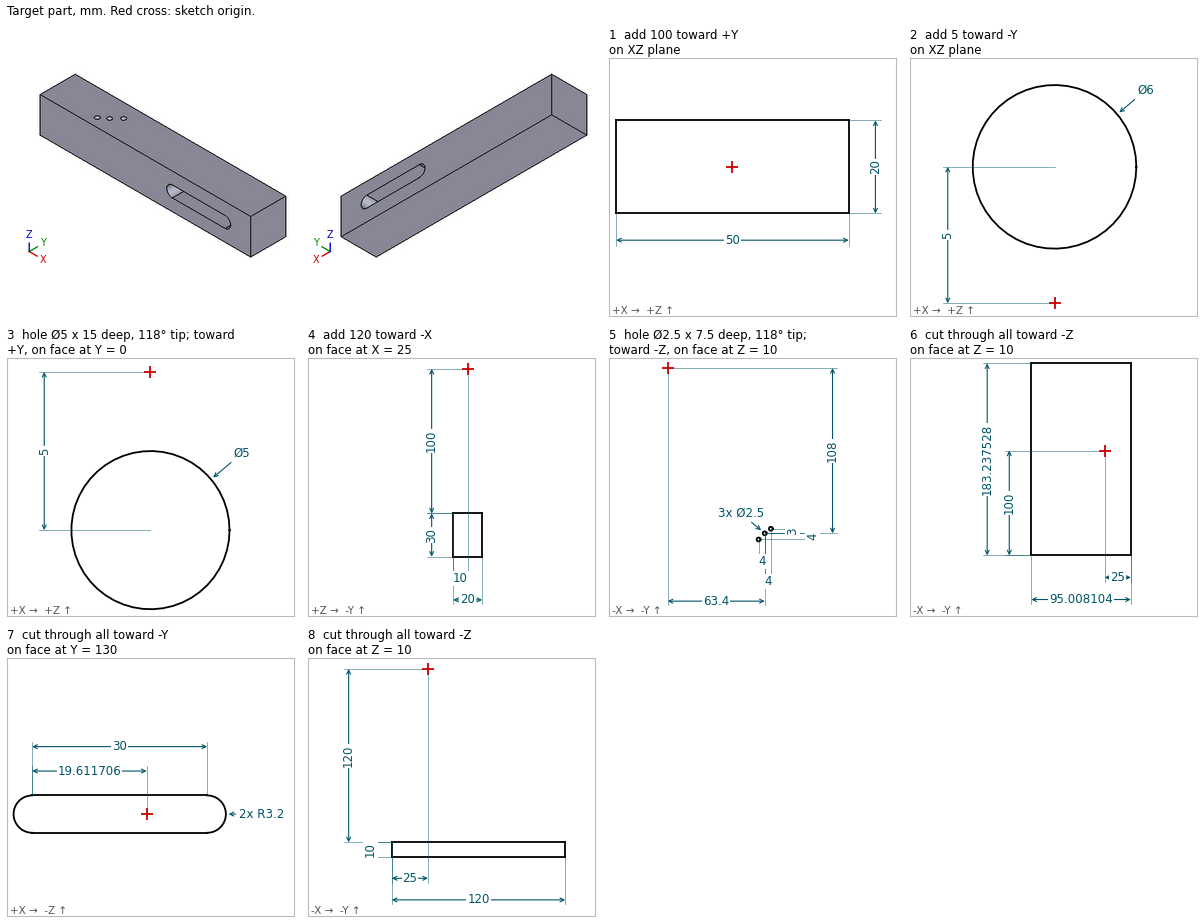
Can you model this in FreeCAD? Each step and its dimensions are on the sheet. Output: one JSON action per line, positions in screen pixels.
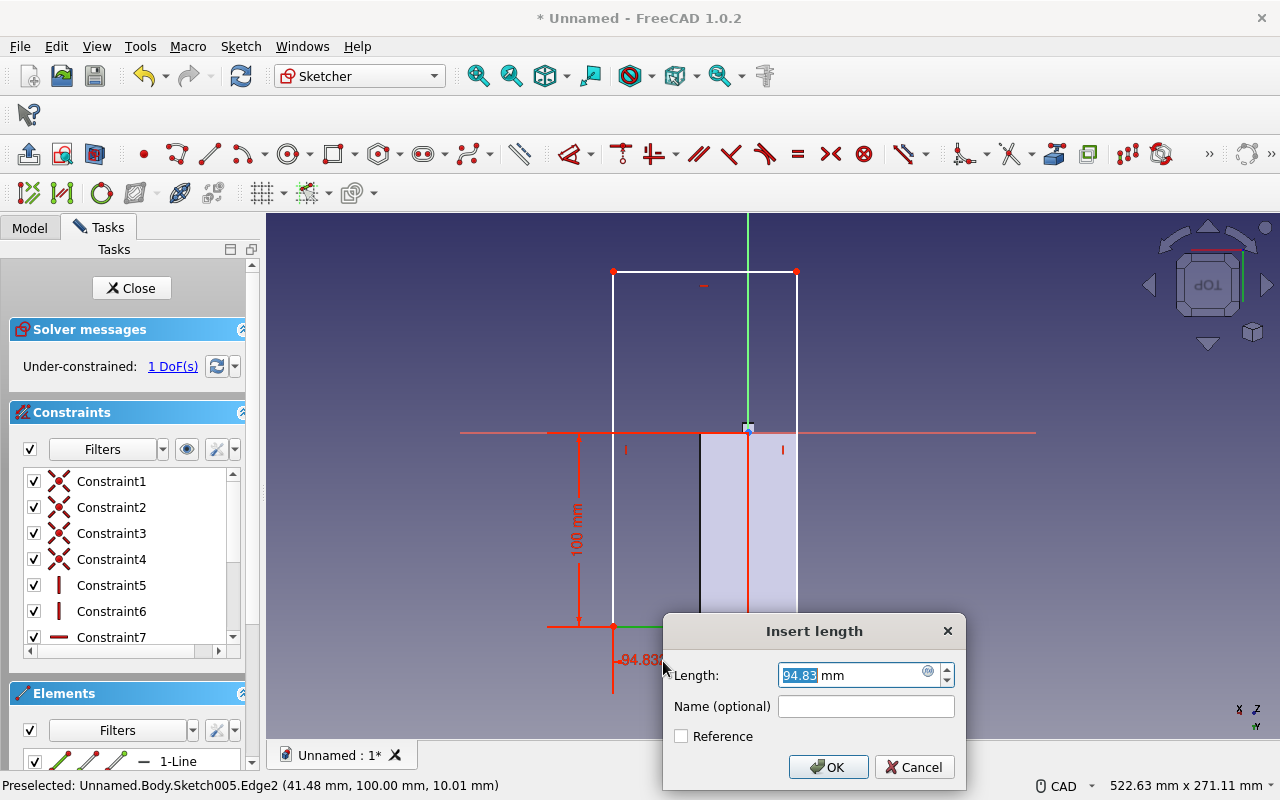
{"action": "type", "text": "95.008104"}
{"action": "key", "text": "Return"}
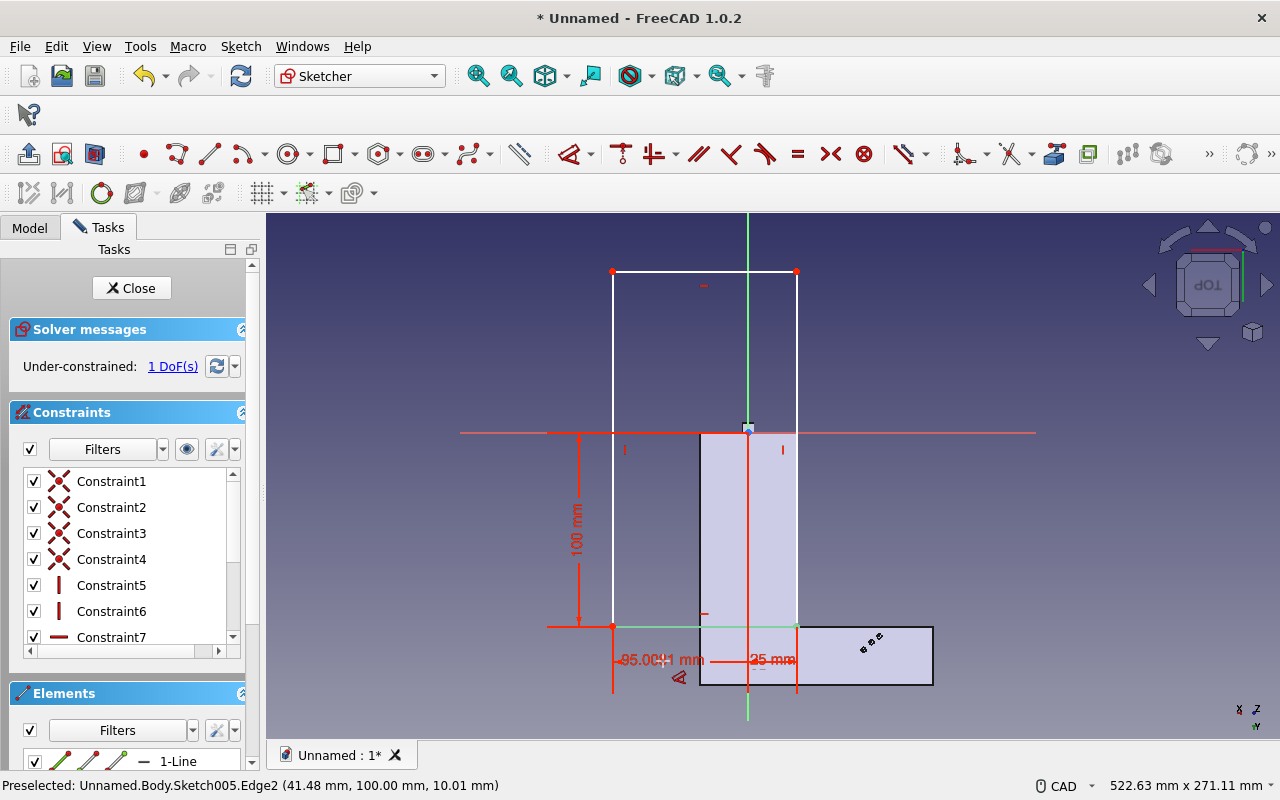
{"action": "left_click", "coordinate": [613, 378]}
{"action": "left_click", "coordinate": [579, 449]}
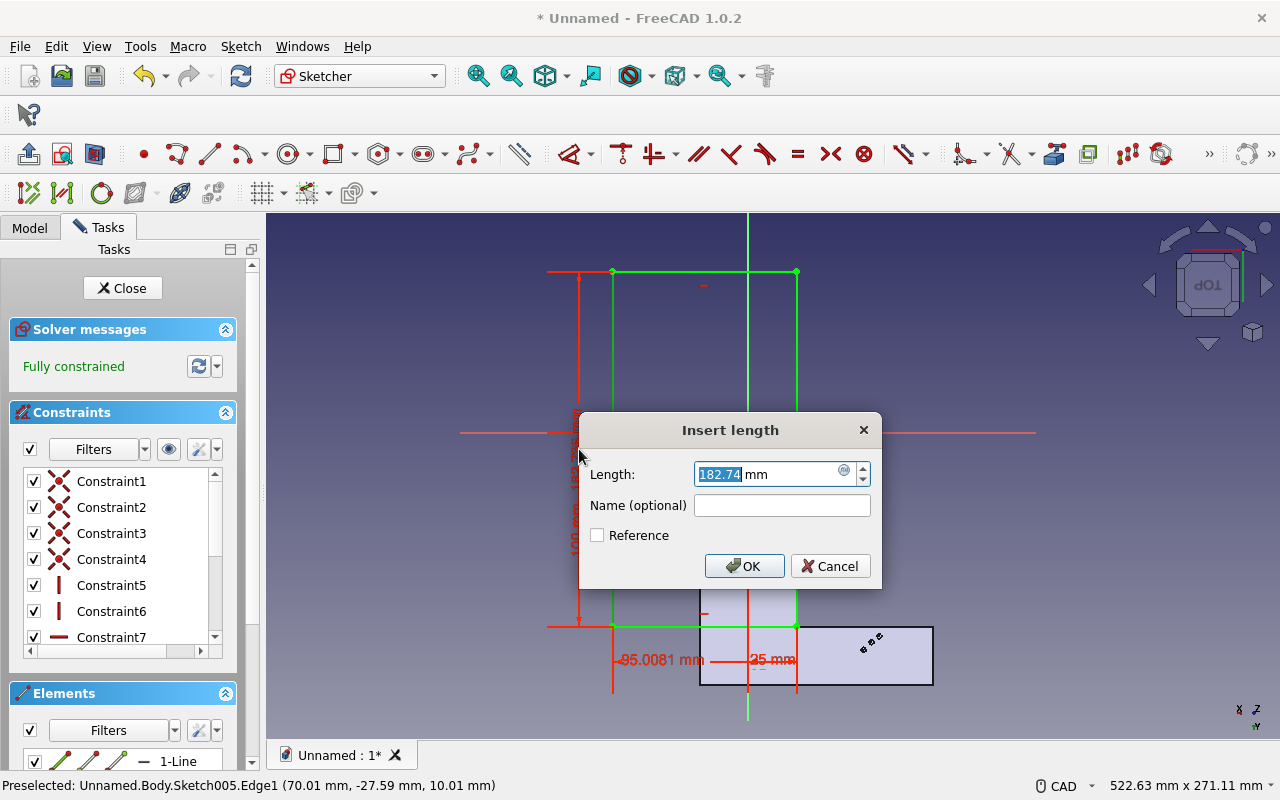
{"action": "type", "text": "183.237528"}
{"action": "key", "text": "Return"}
{"action": "key", "text": "Escape"}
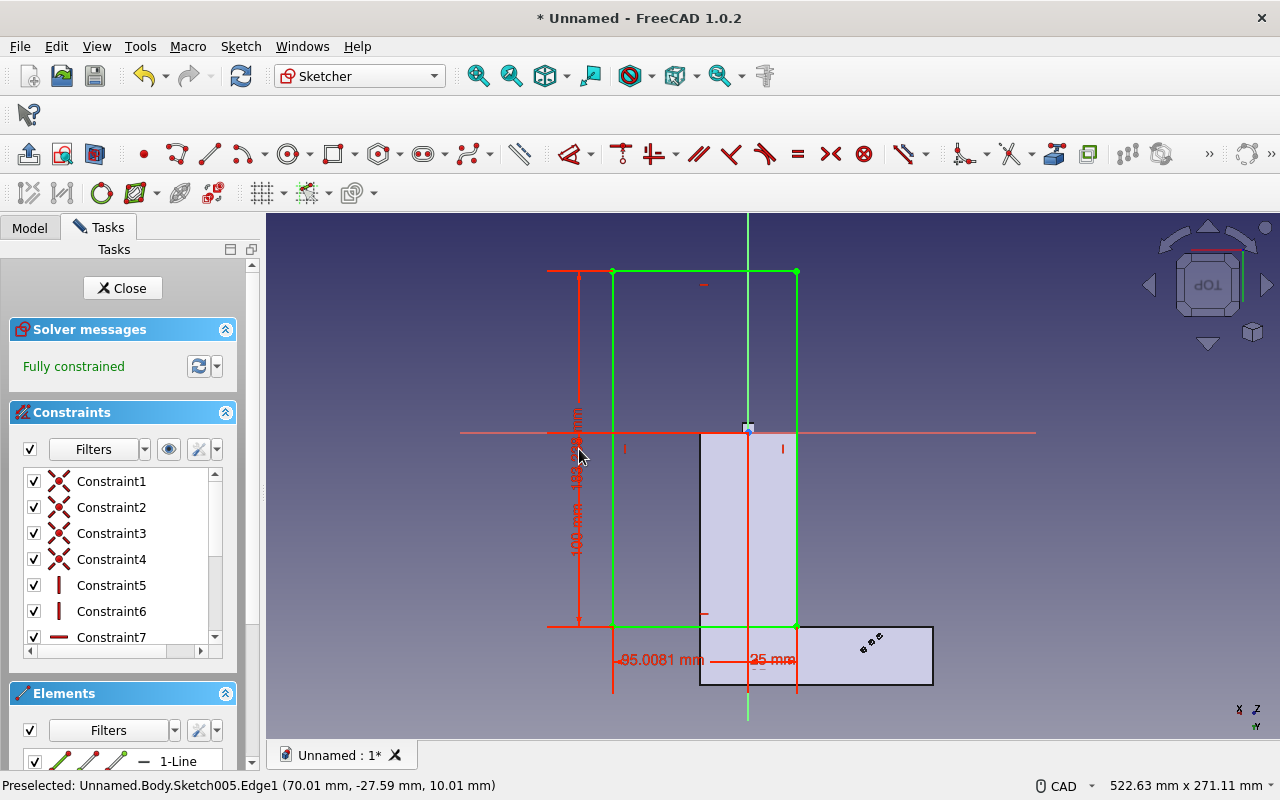
{"action": "left_click", "coordinate": [123, 288]}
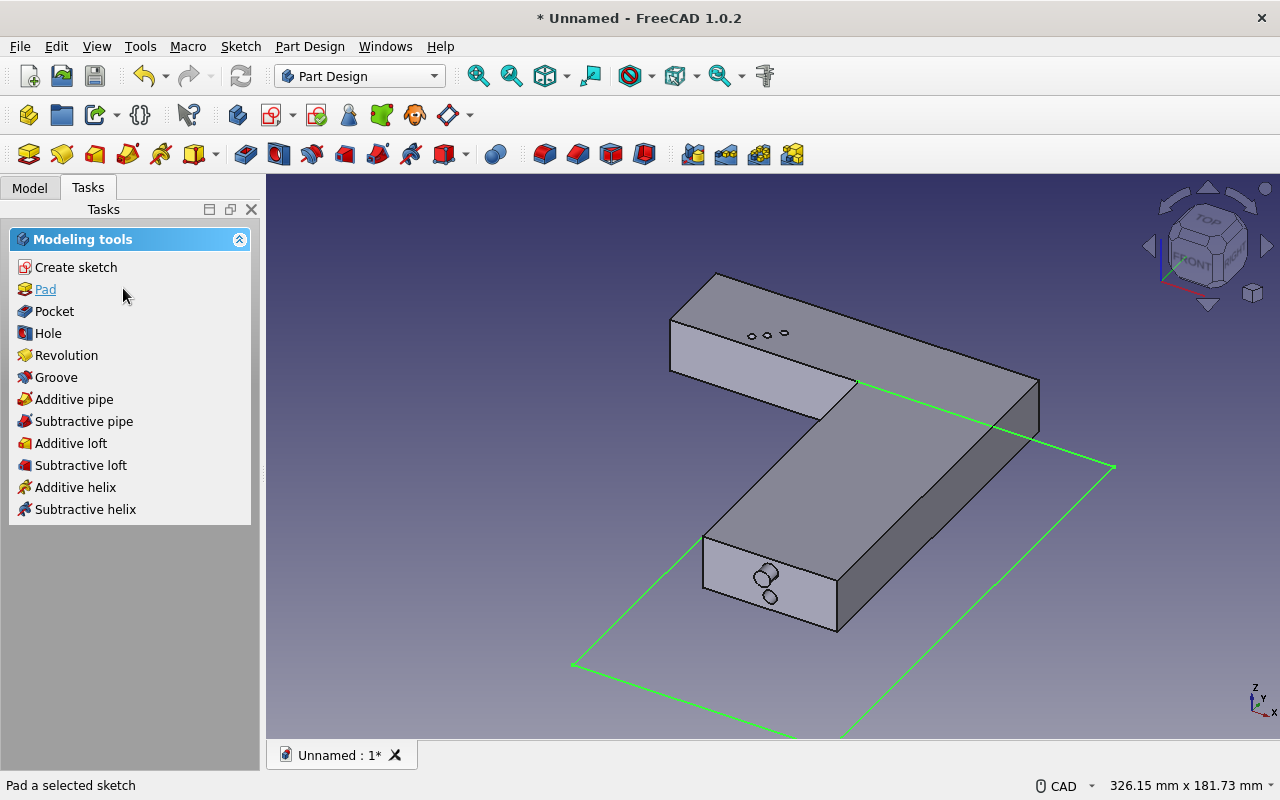
{"action": "left_click", "coordinate": [246, 154]}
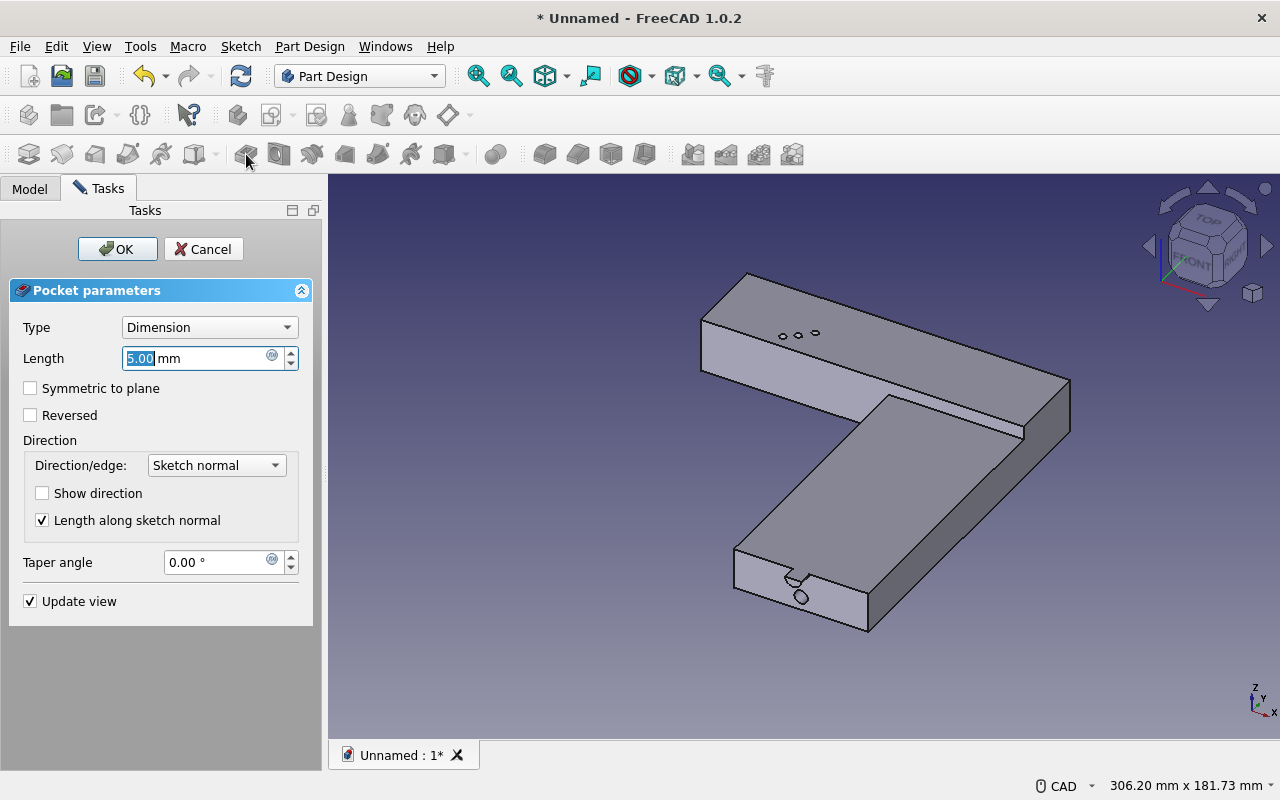
{"action": "left_click", "coordinate": [210, 328]}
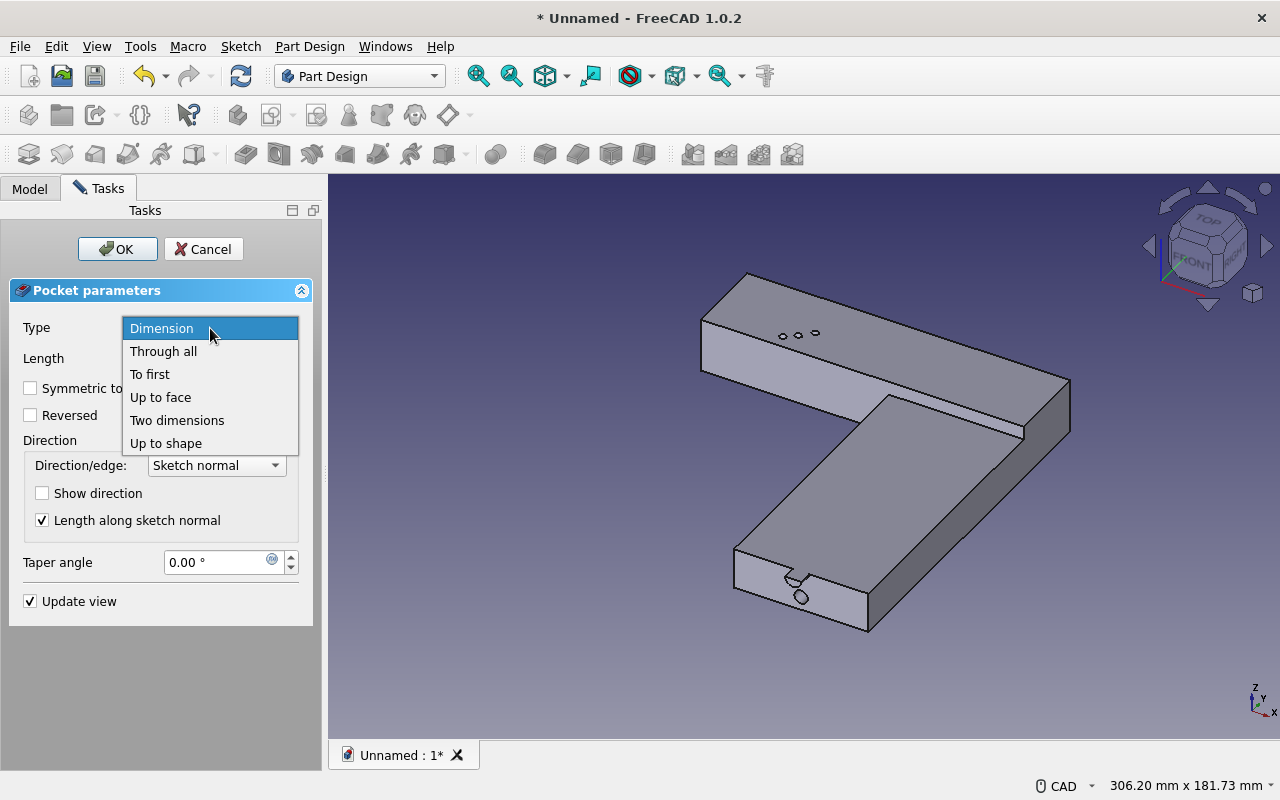
{"action": "left_click", "coordinate": [208, 352]}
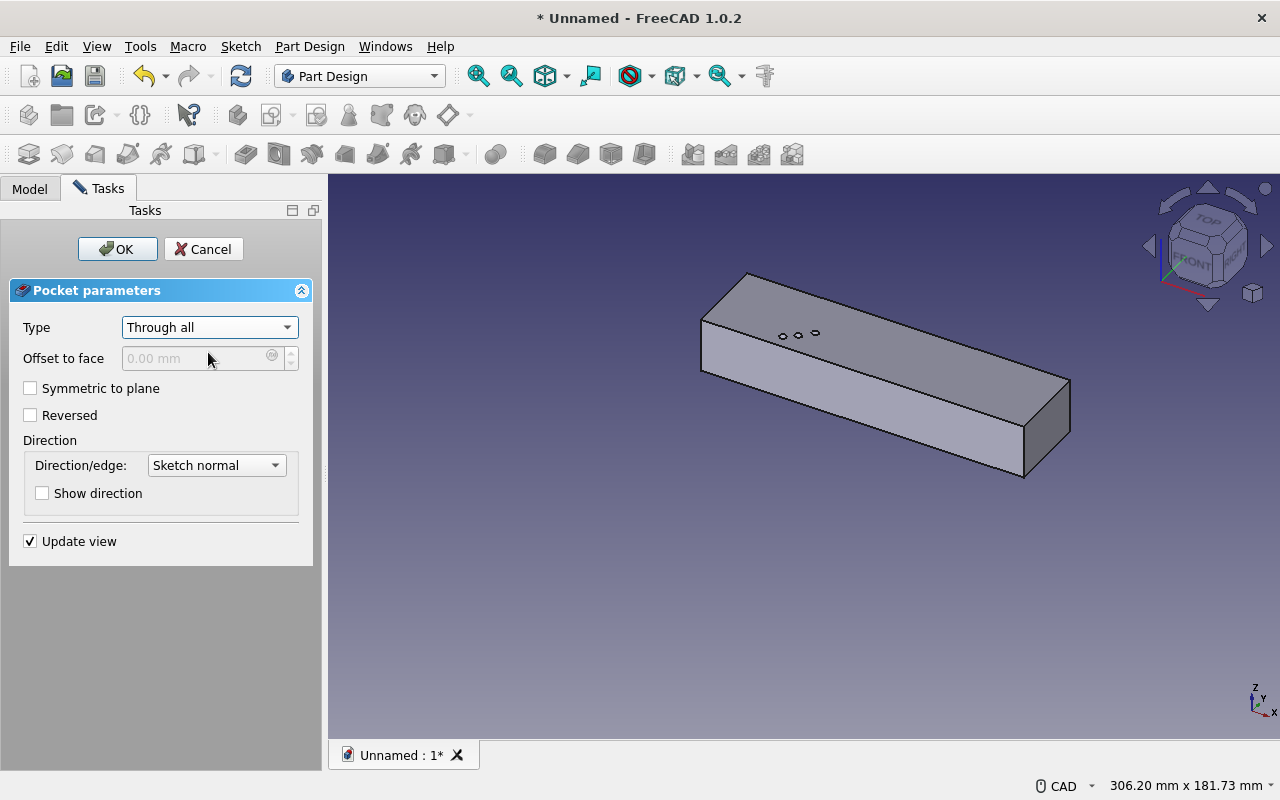
{"action": "left_click", "coordinate": [118, 249]}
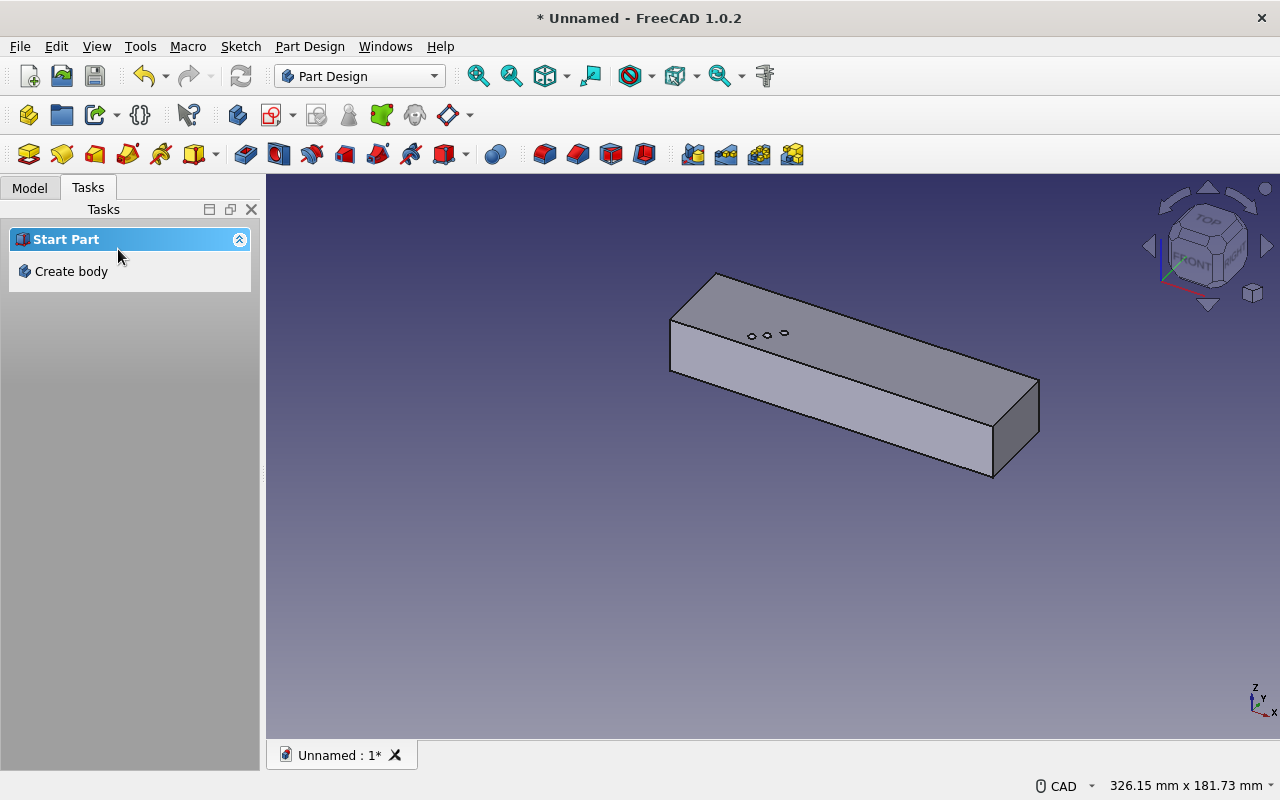
{"action": "key", "text": "v f"}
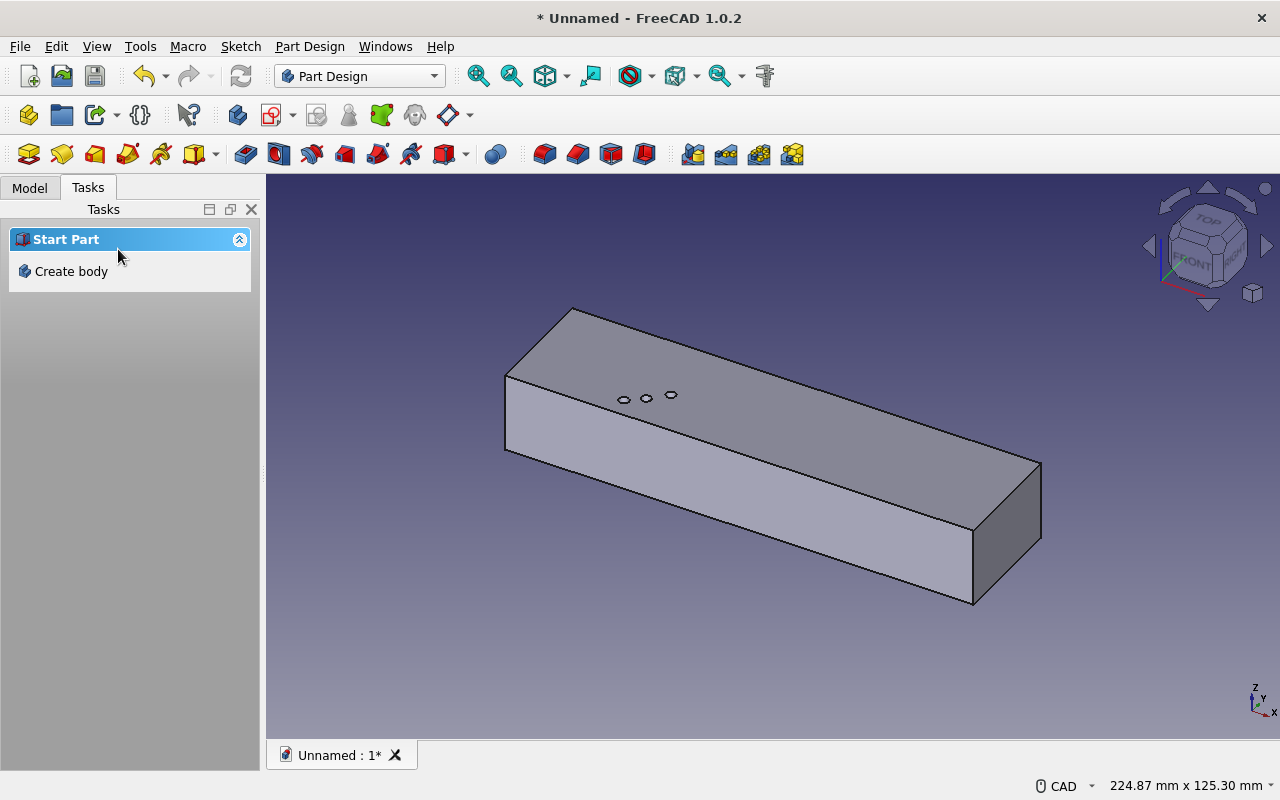
{"action": "key", "text": "4"}